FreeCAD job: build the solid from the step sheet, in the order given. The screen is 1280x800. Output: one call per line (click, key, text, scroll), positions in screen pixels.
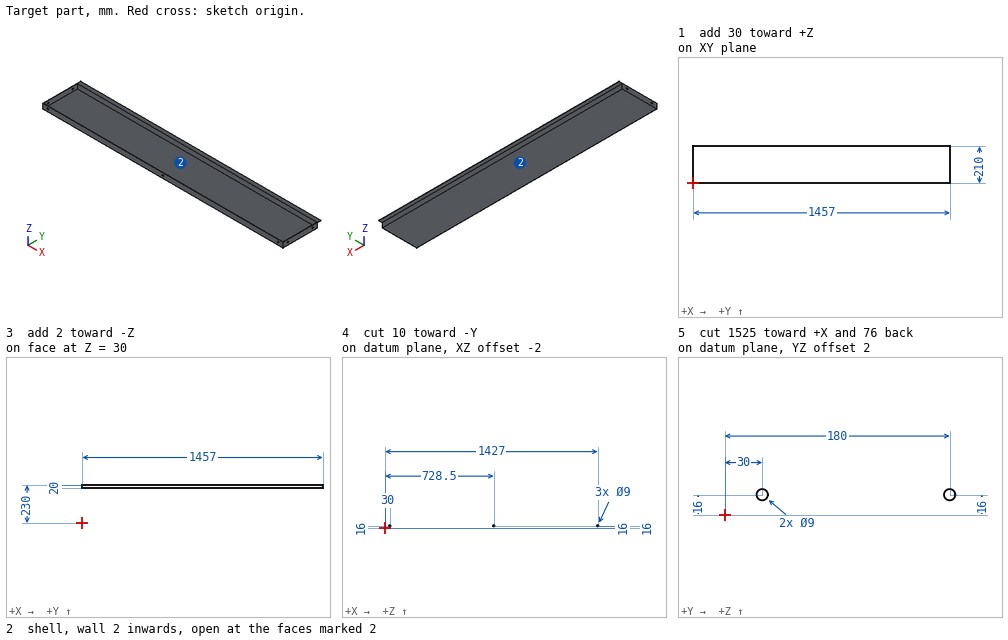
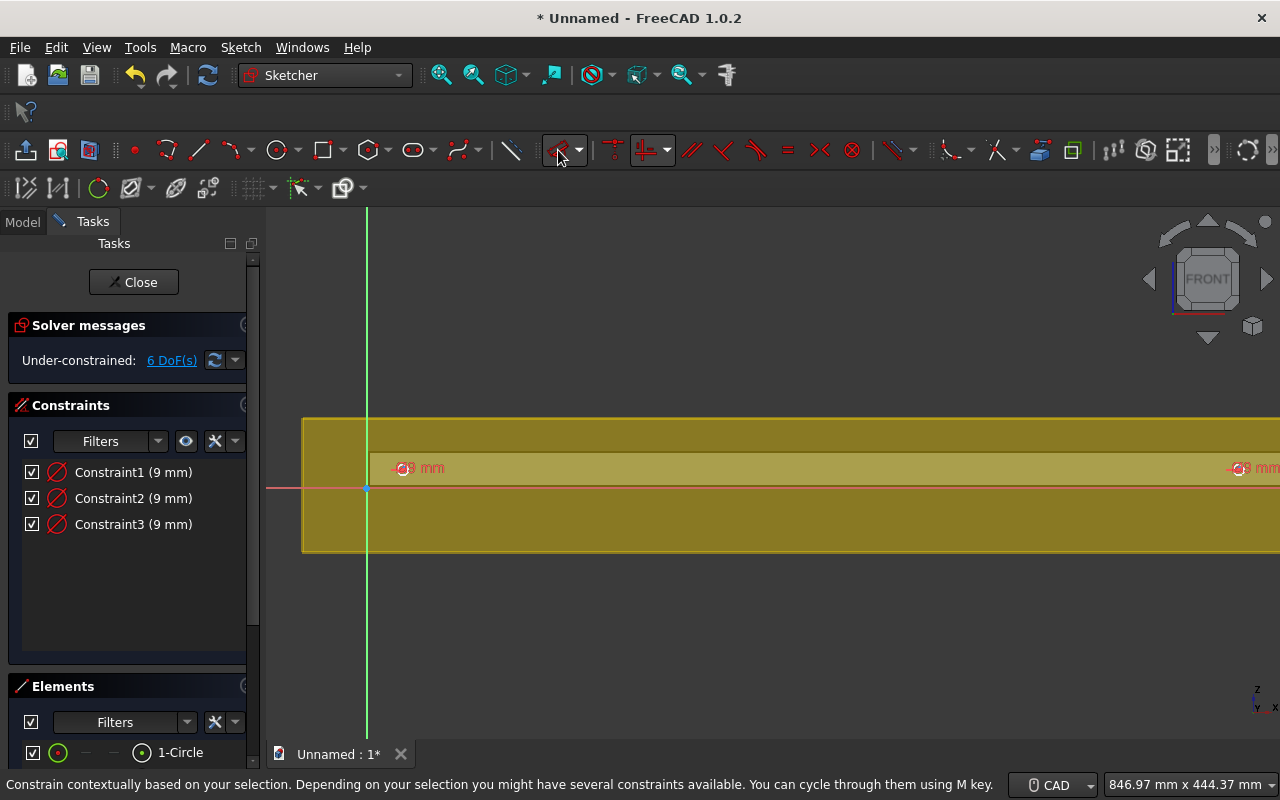
scroll(402, 471, down, 5)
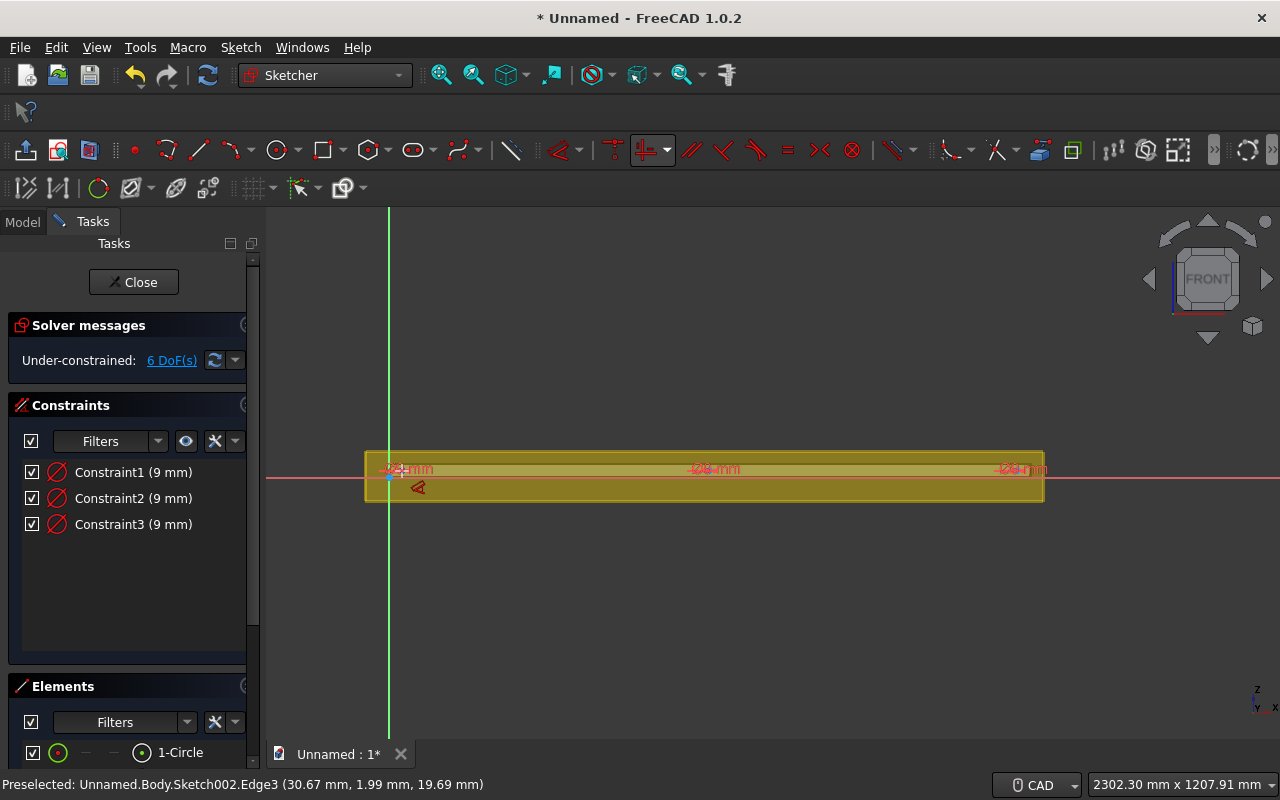
scroll(1017, 471, up, 9)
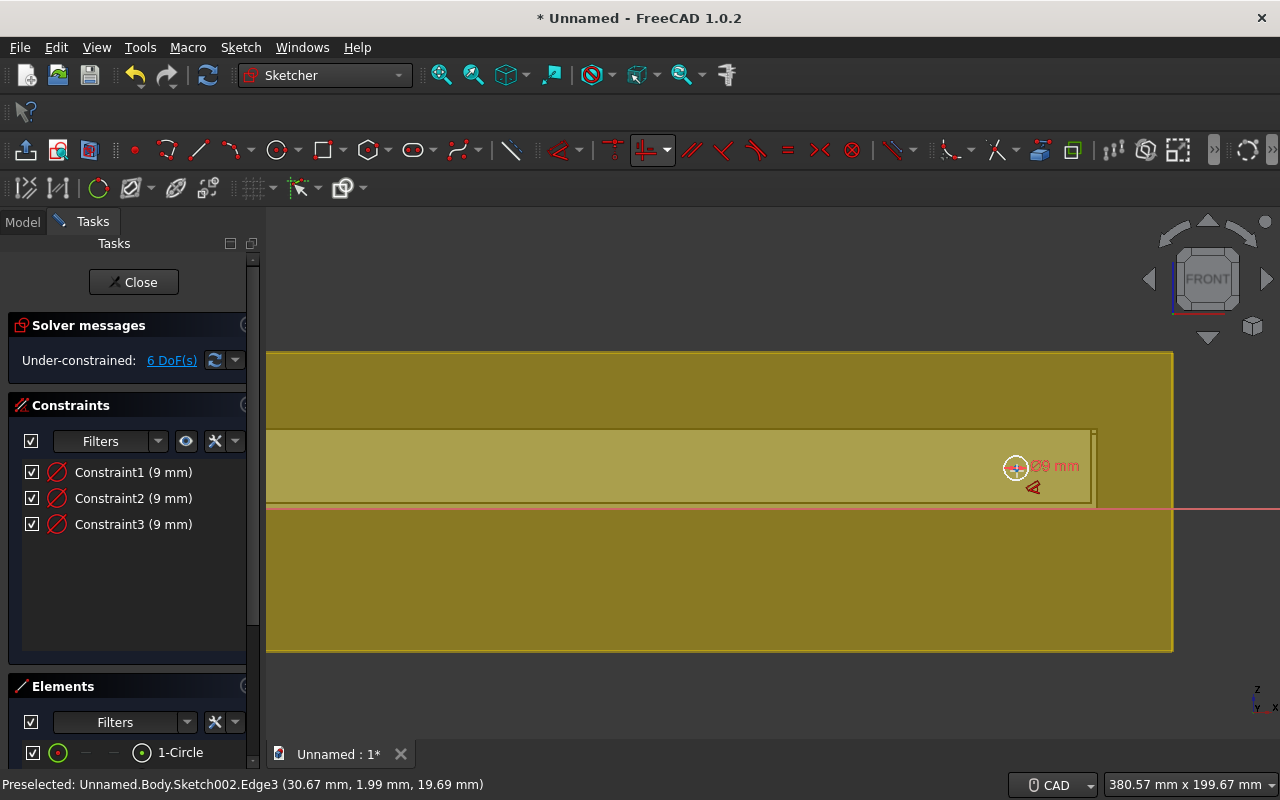
click(1016, 468)
click(1050, 488)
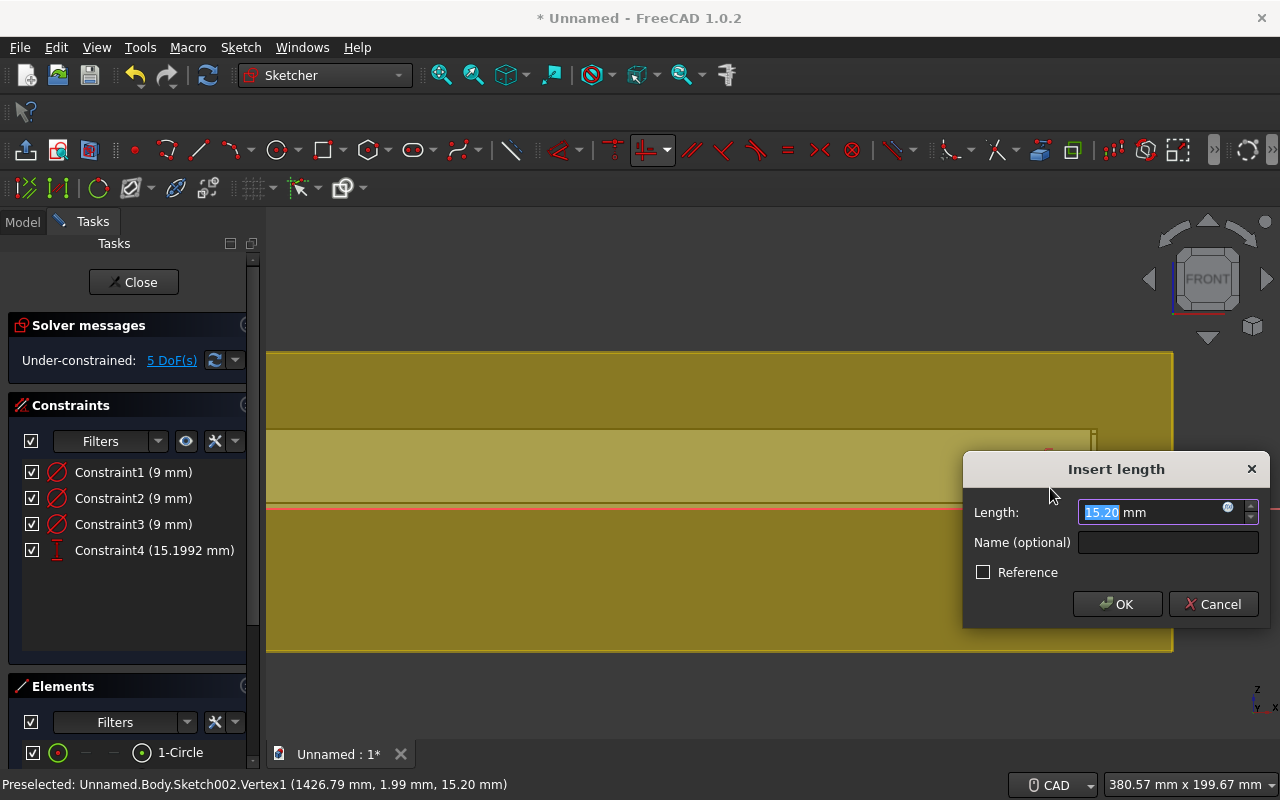
text(16)
key(Return)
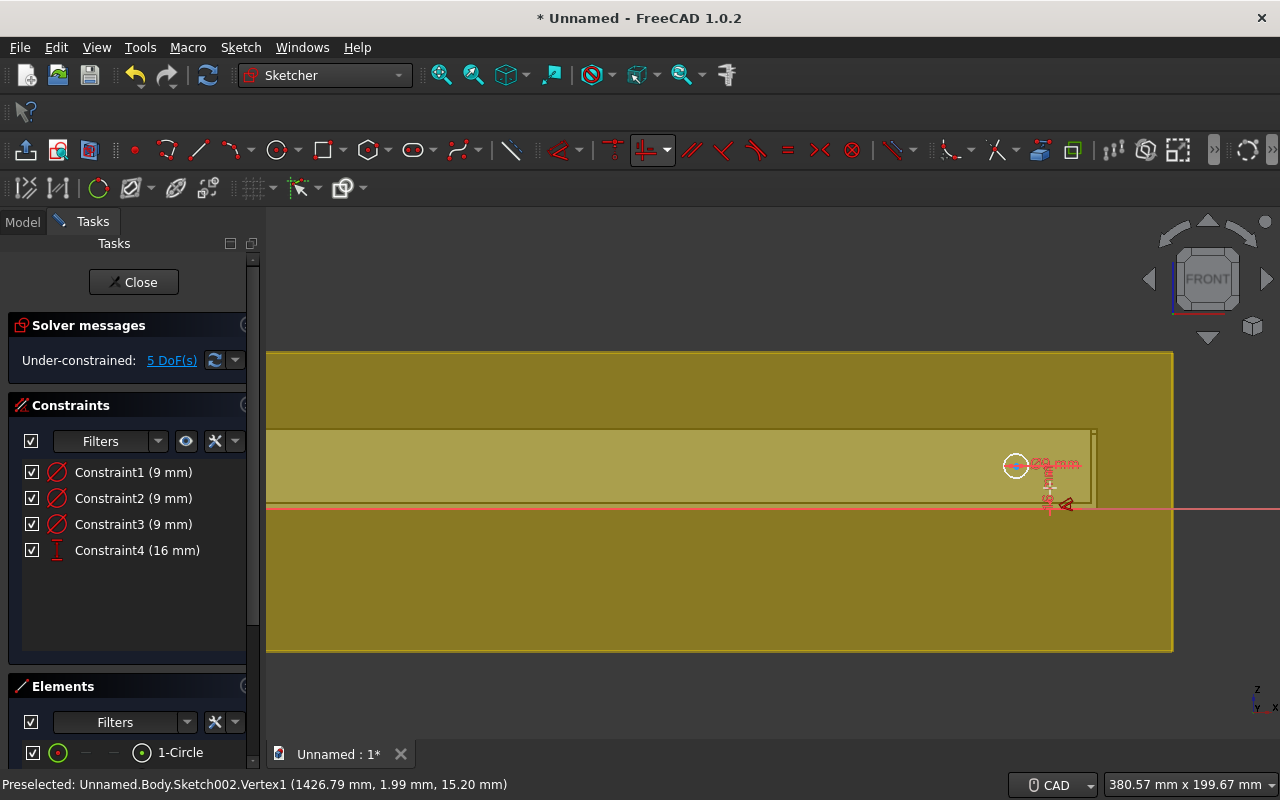
scroll(1018, 471, down, 9)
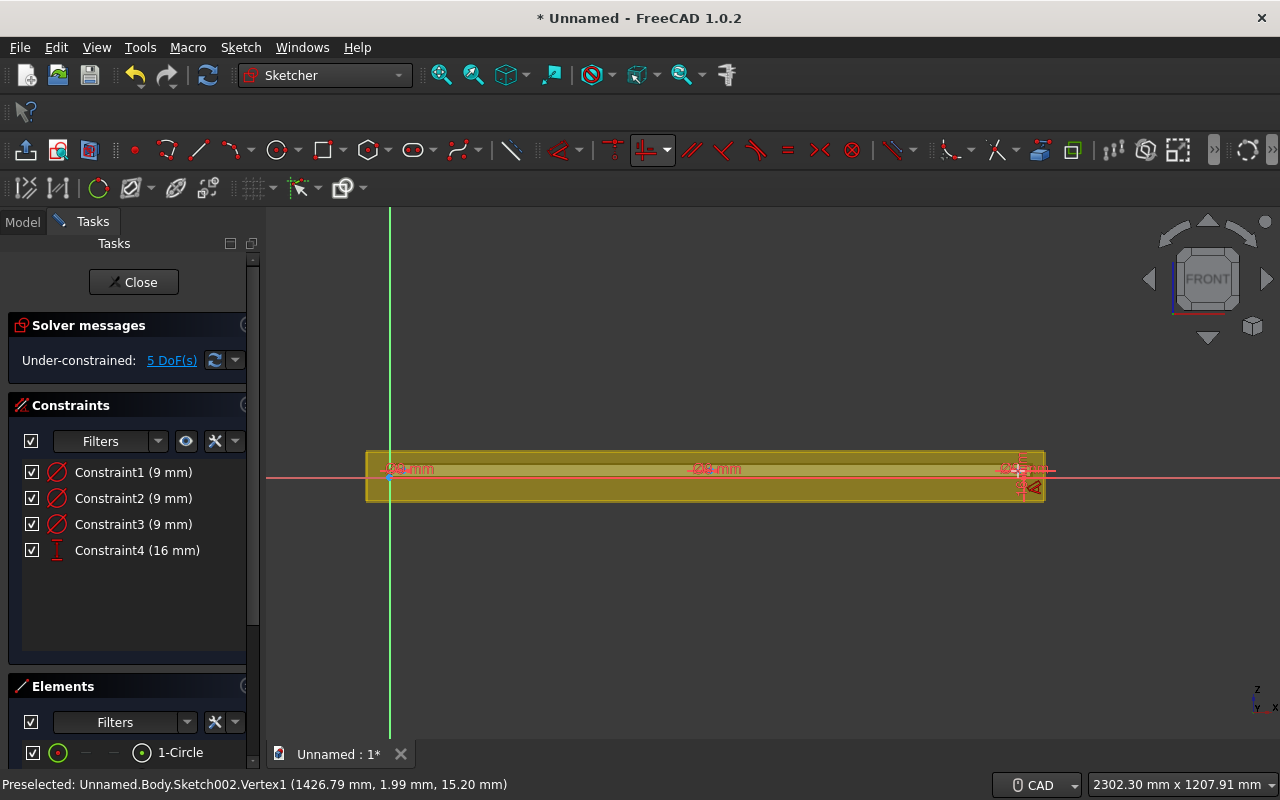
scroll(711, 471, up, 9)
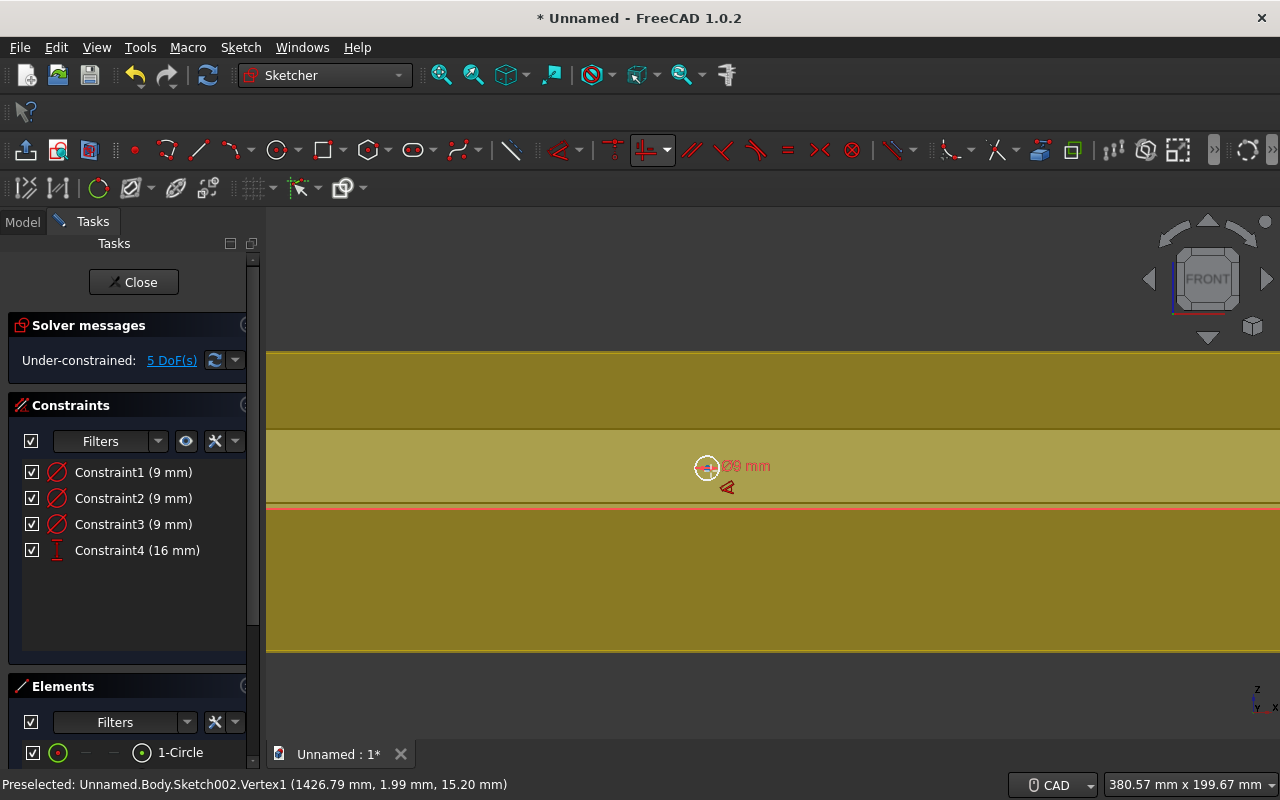
click(707, 468)
click(741, 488)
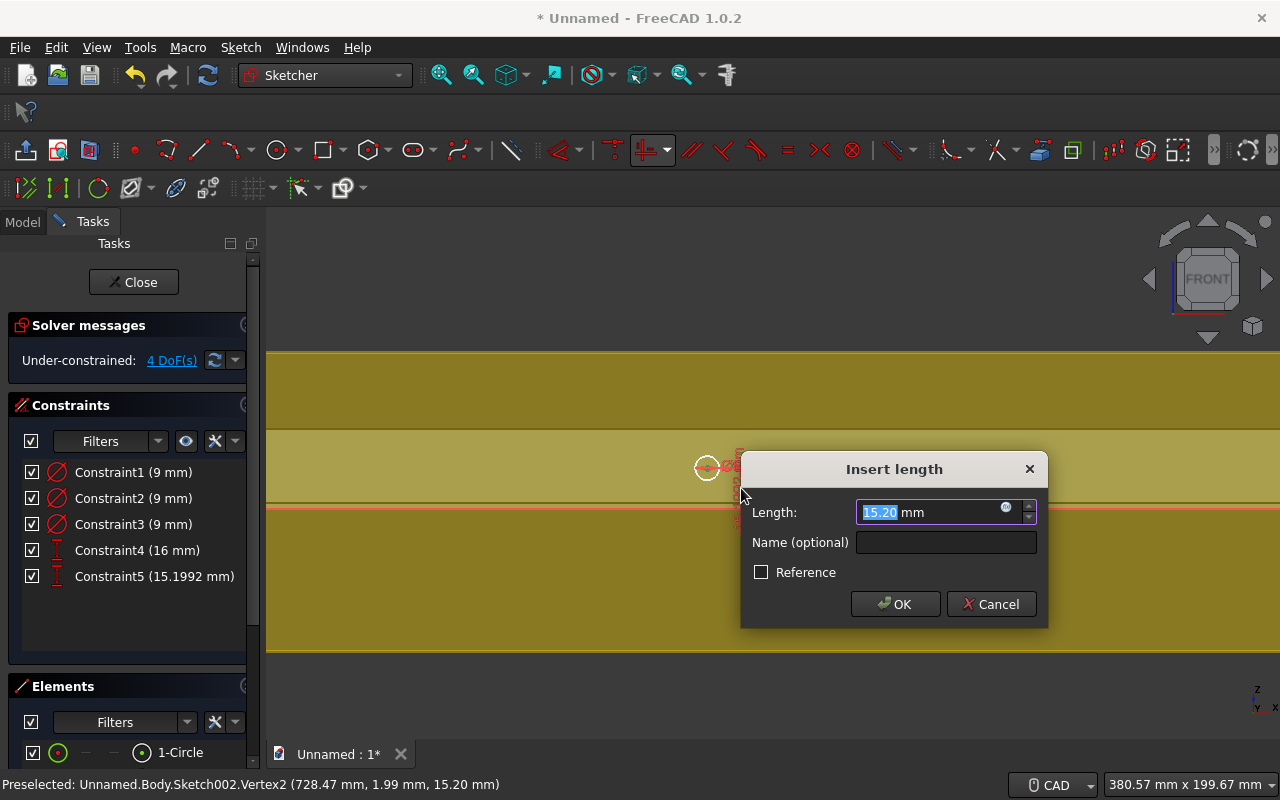
text(16)
key(Return)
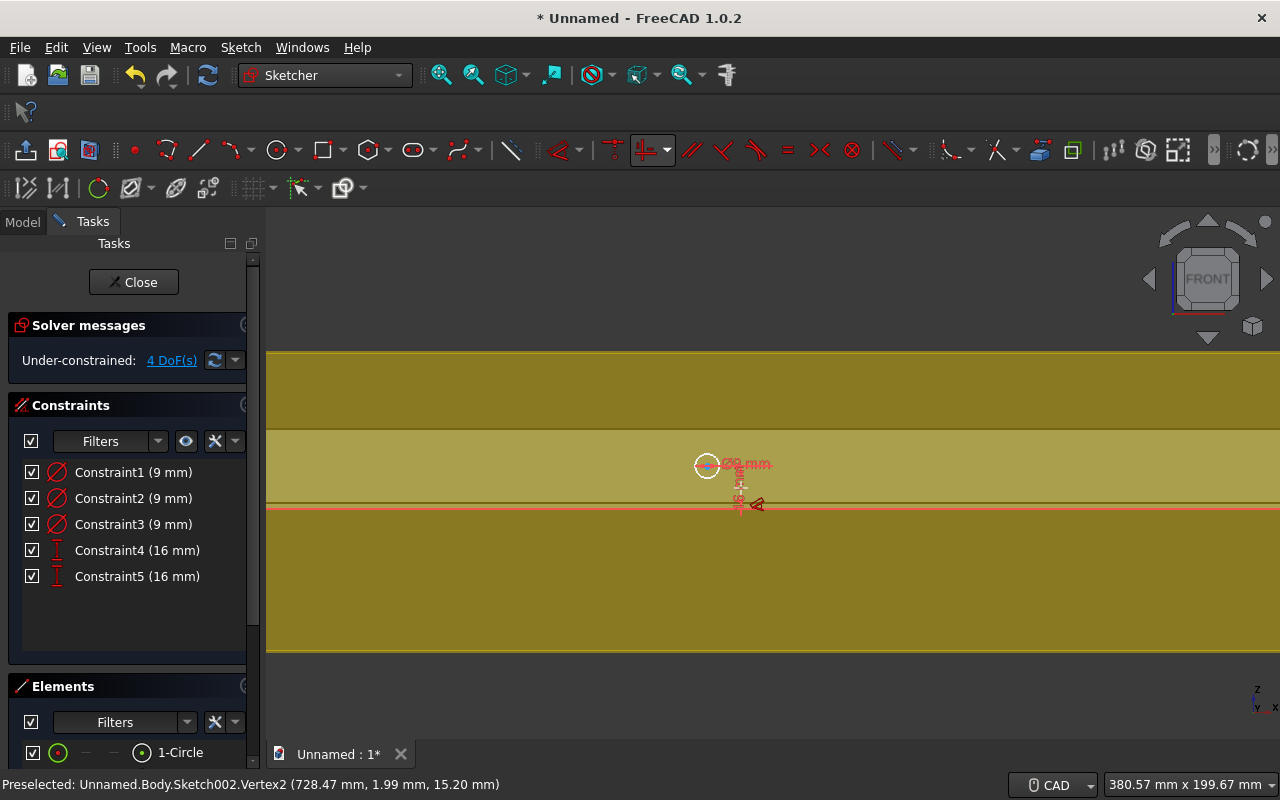
scroll(711, 471, down, 9)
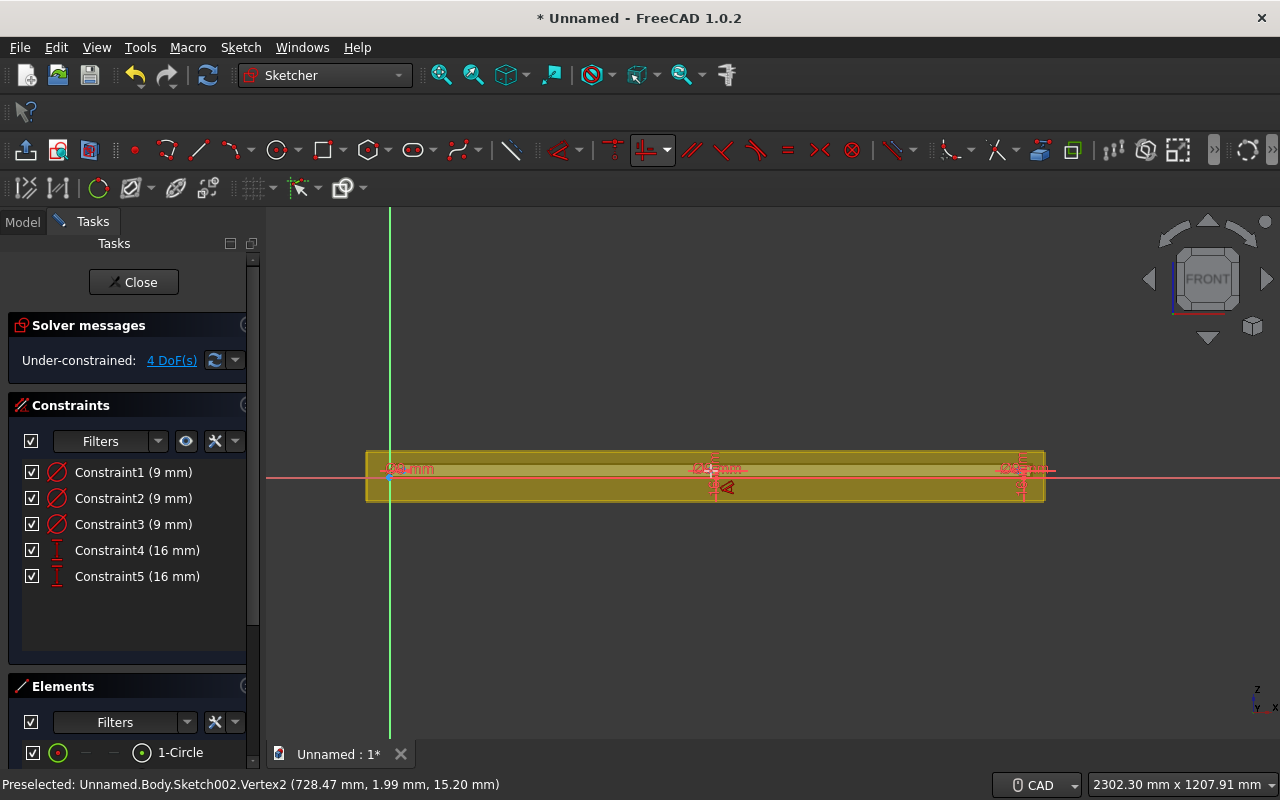
scroll(403, 471, up, 6)